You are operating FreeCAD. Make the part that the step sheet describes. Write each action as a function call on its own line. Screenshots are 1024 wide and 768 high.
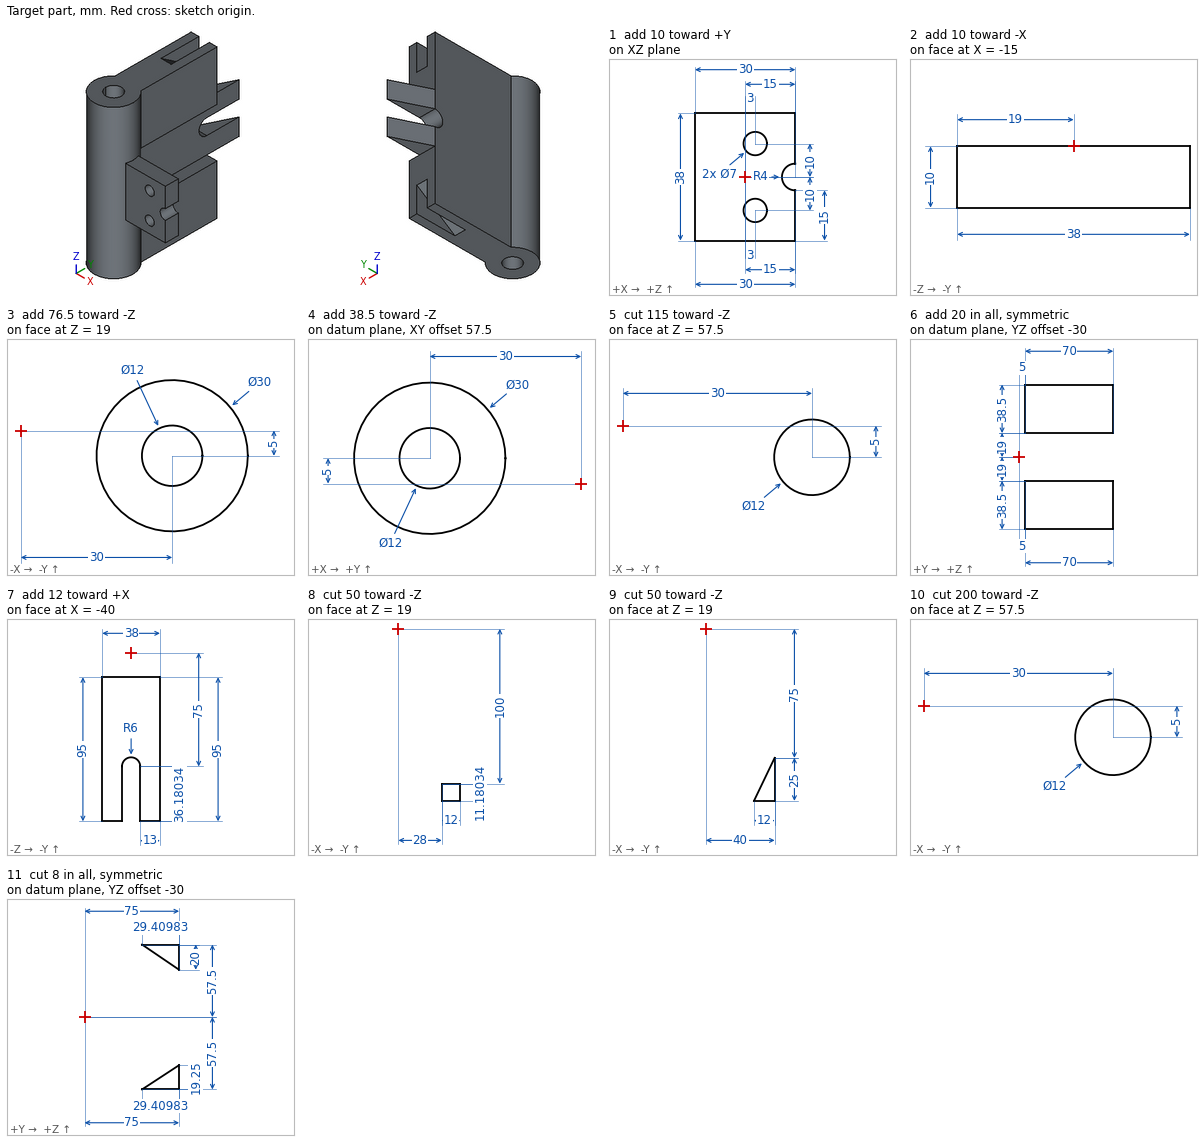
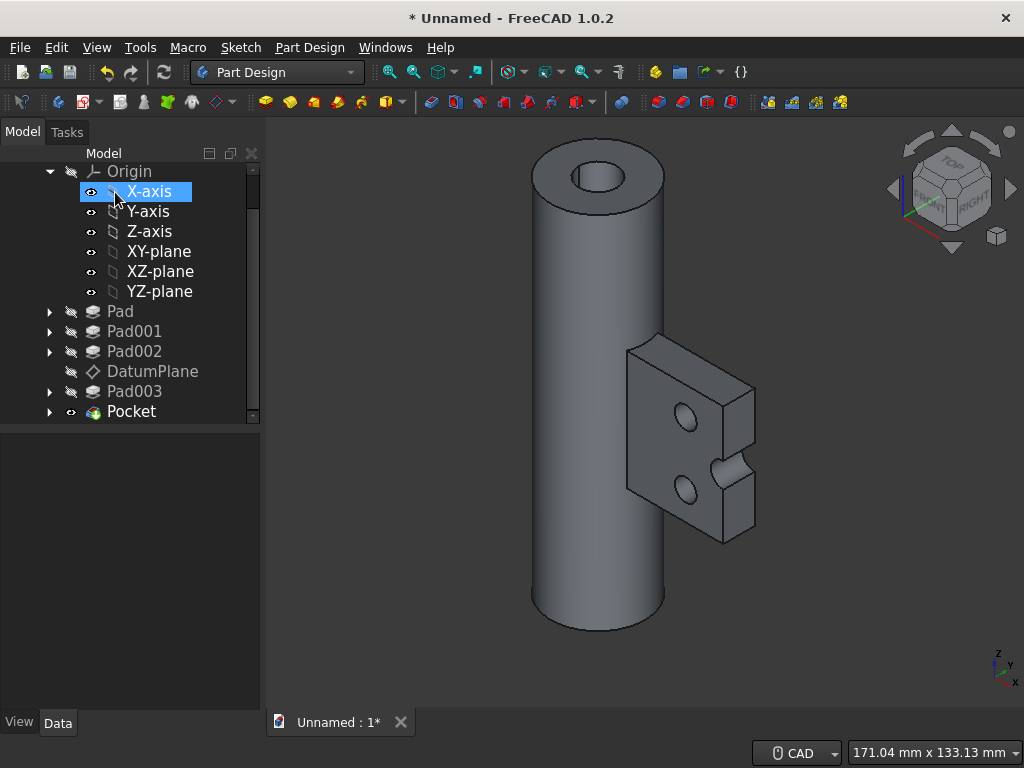
click(136, 292)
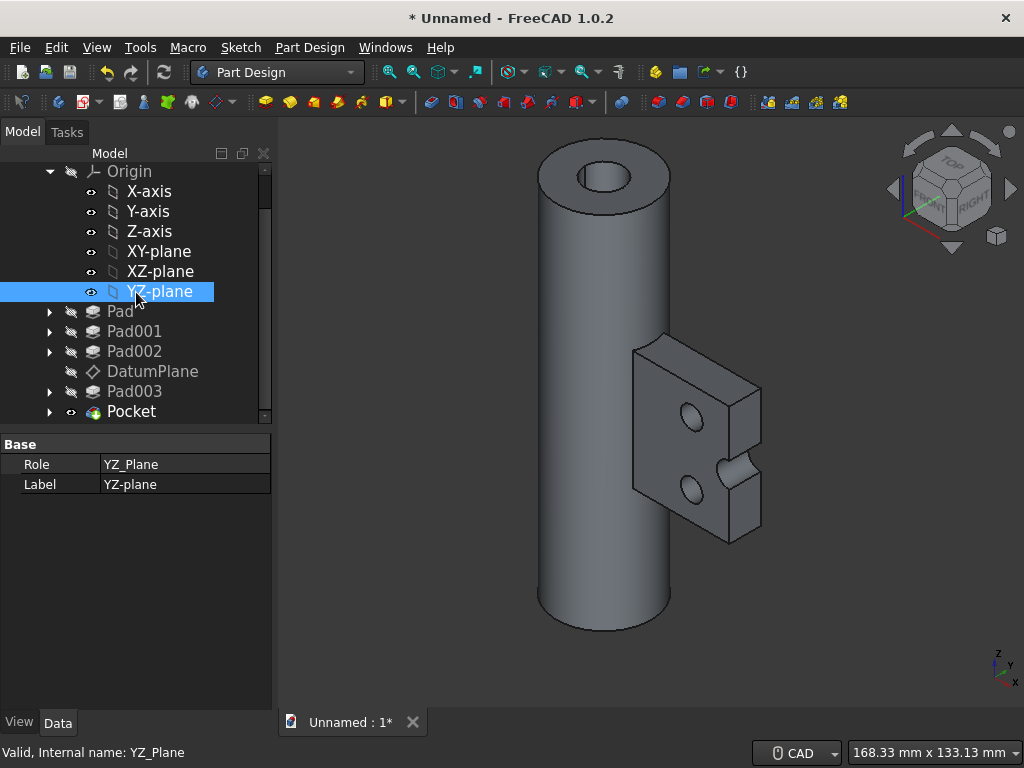
click(216, 102)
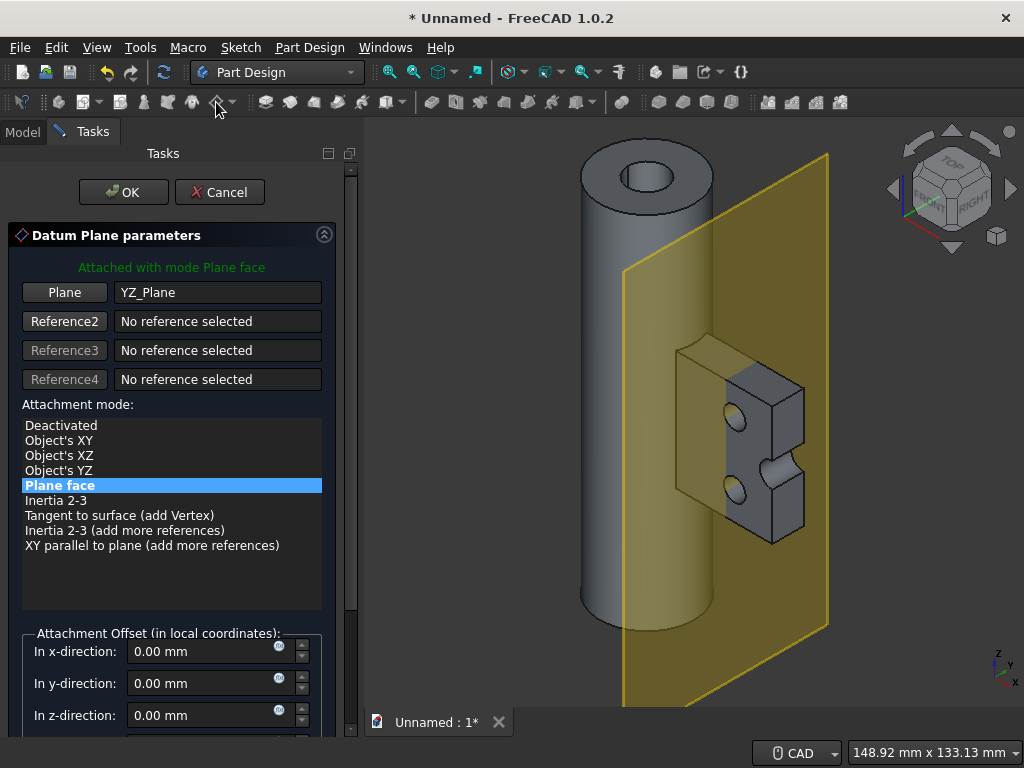
triple_click(210, 715)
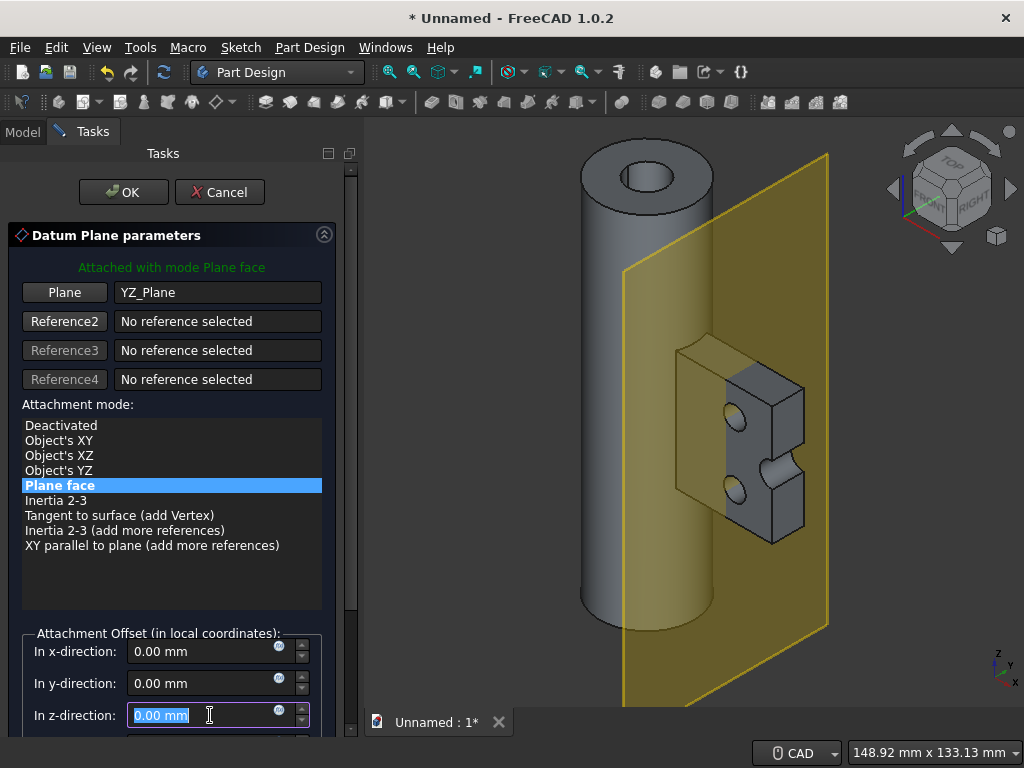
text(-30)
key(Tab)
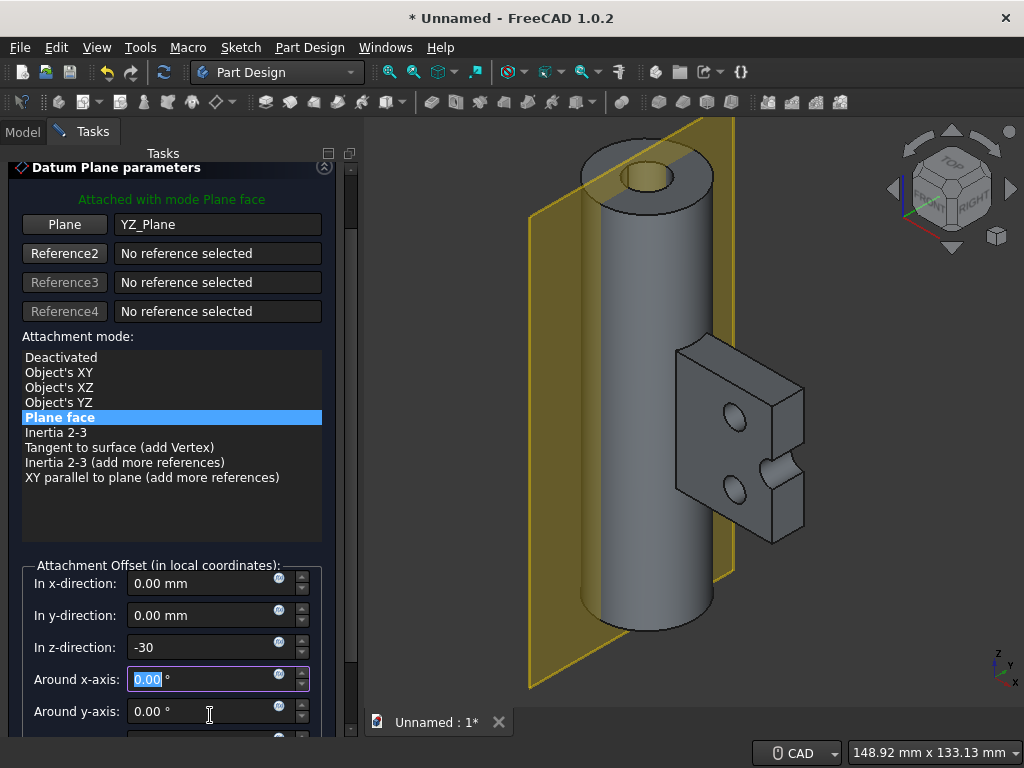
scroll(351, 450, up, 2)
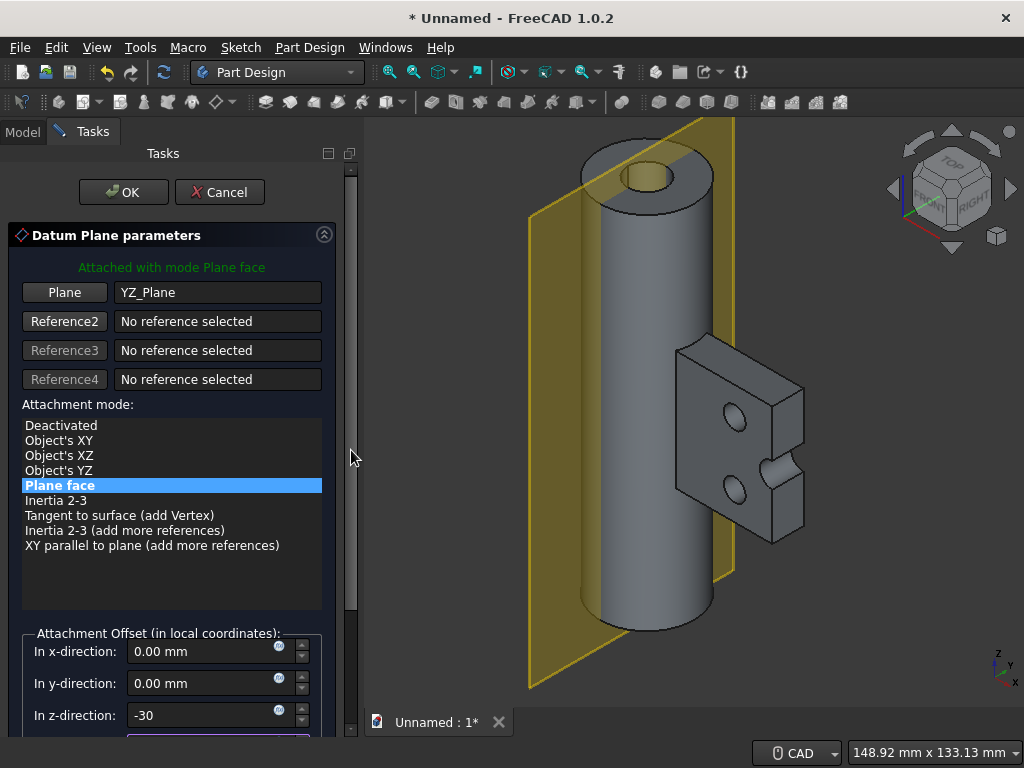
click(124, 192)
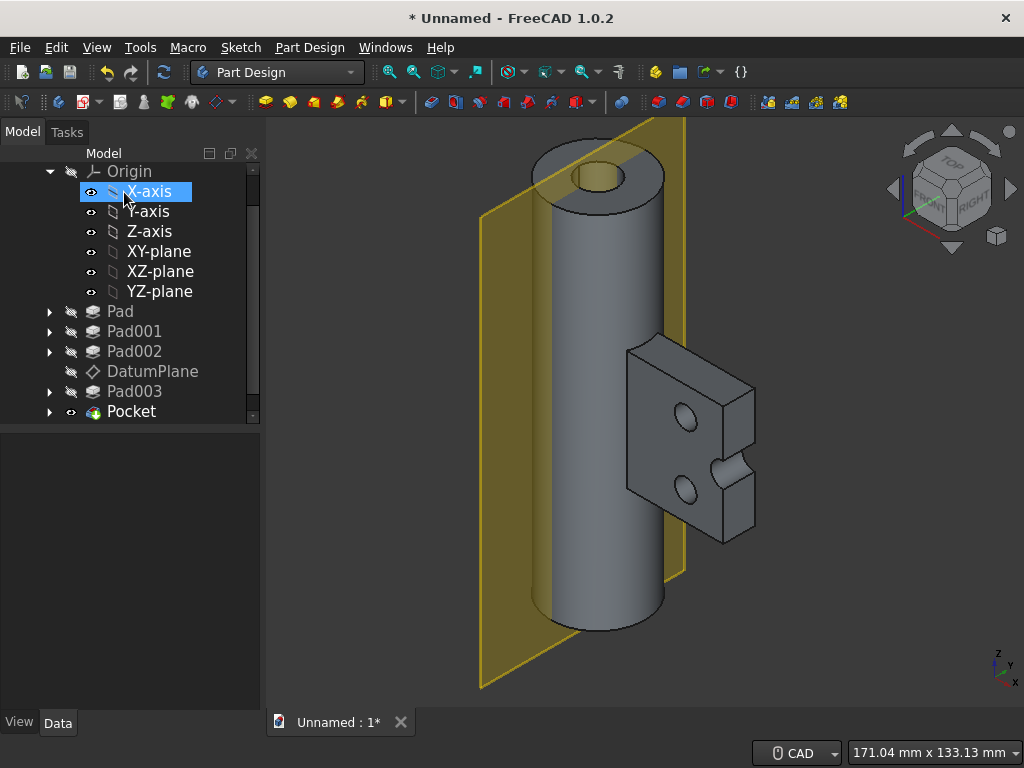
scroll(140, 287, down, 3)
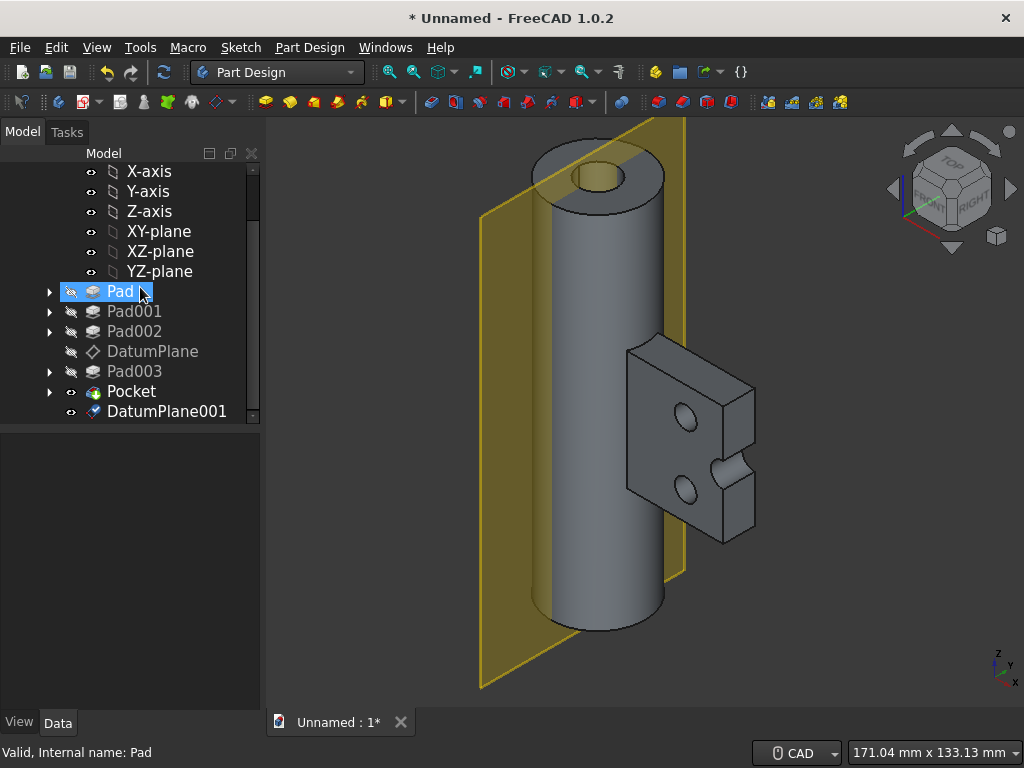
click(116, 412)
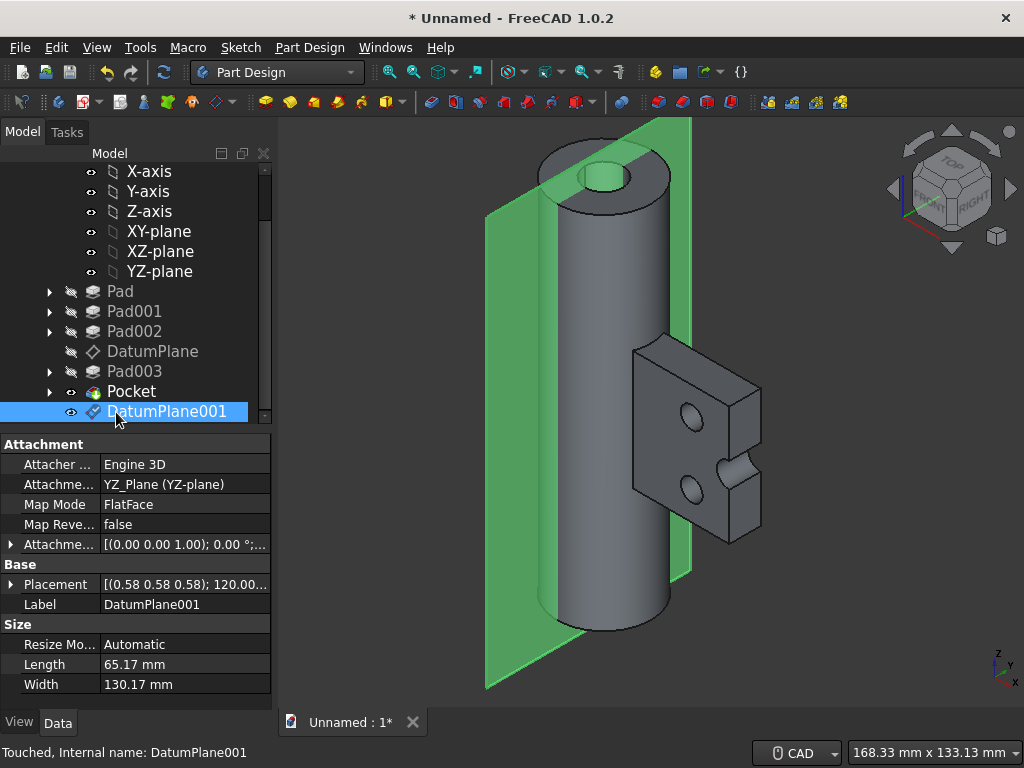
click(84, 102)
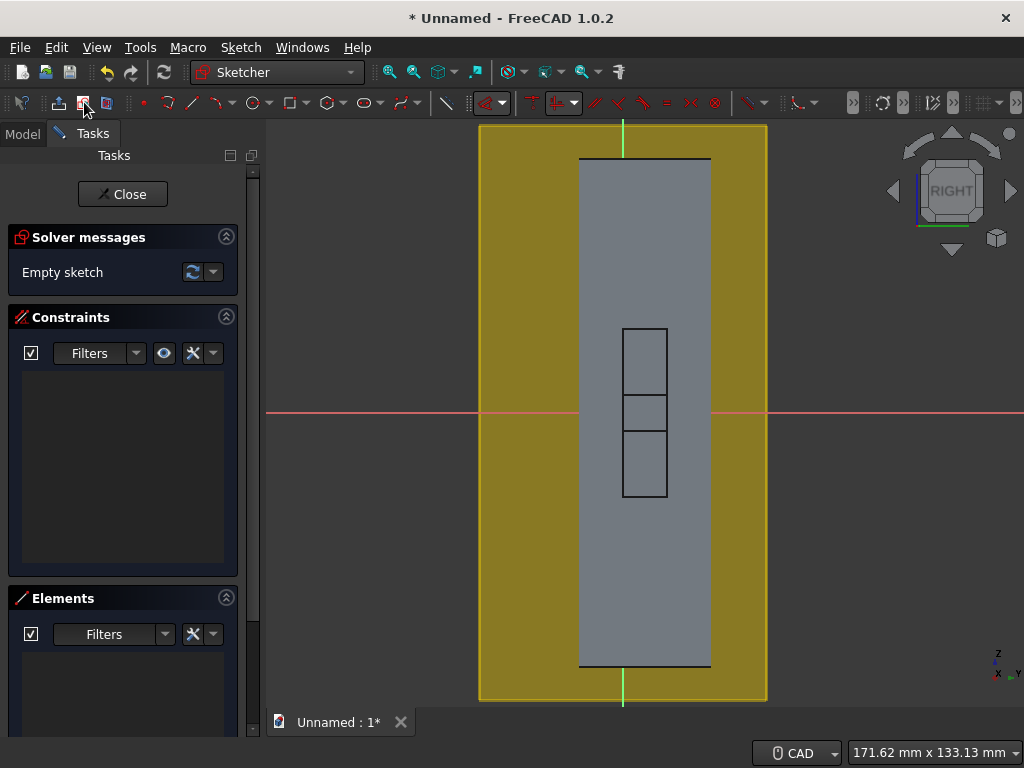
click(108, 104)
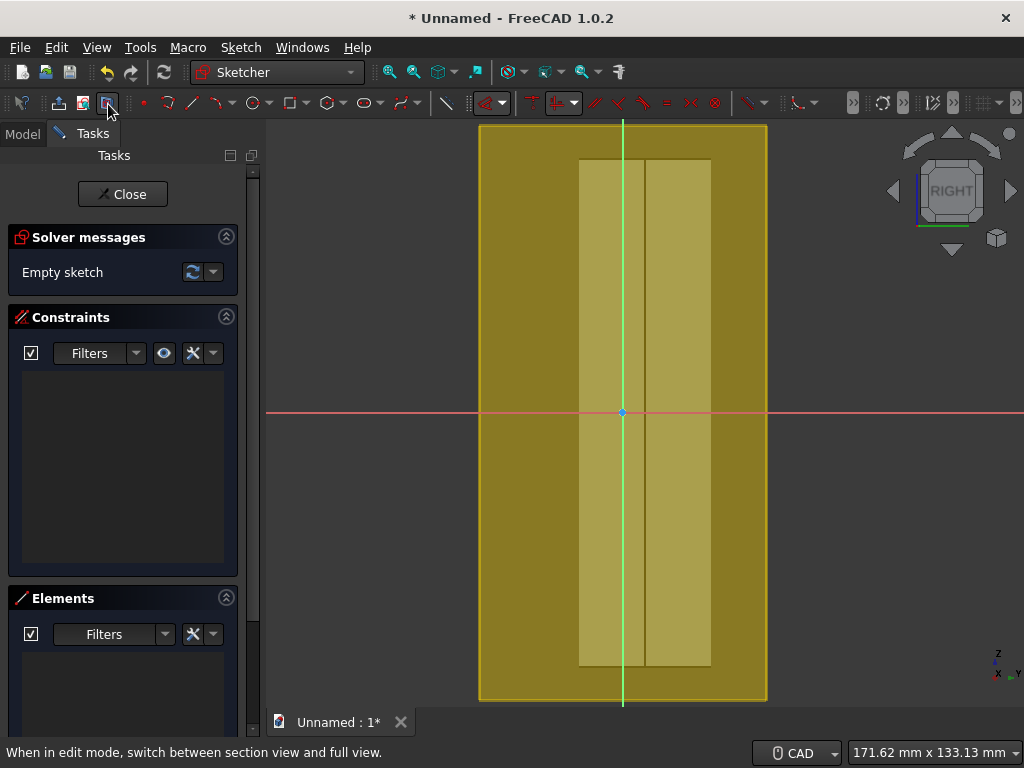
scroll(294, 413, down, 2)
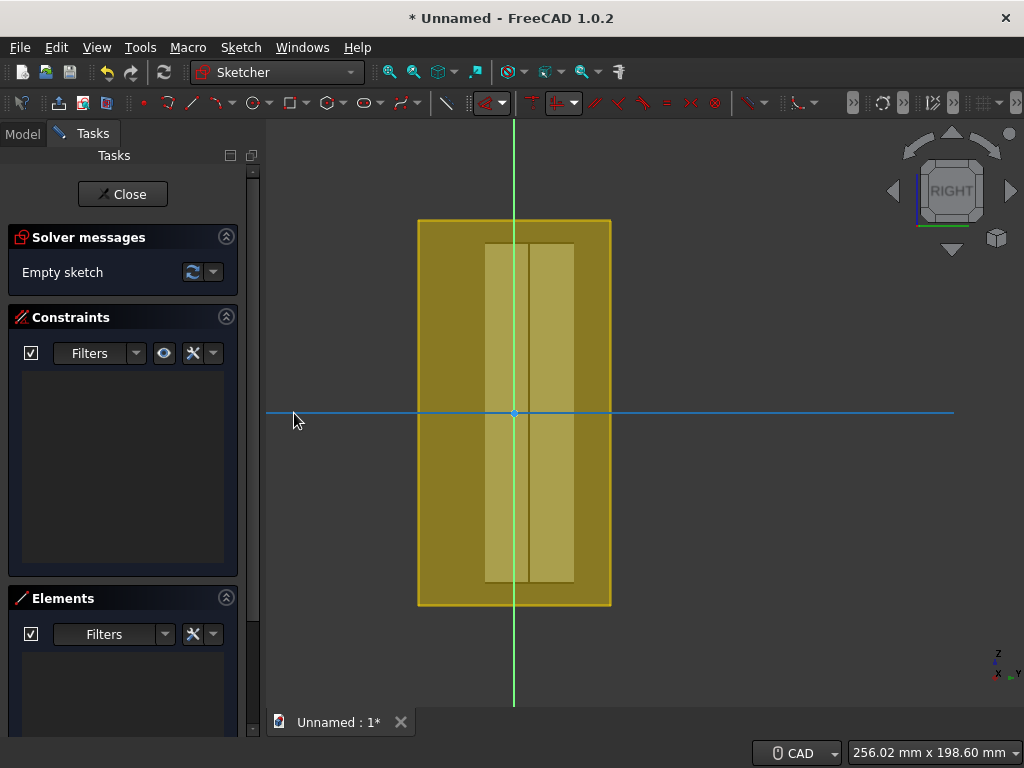
key(g)
key(r)